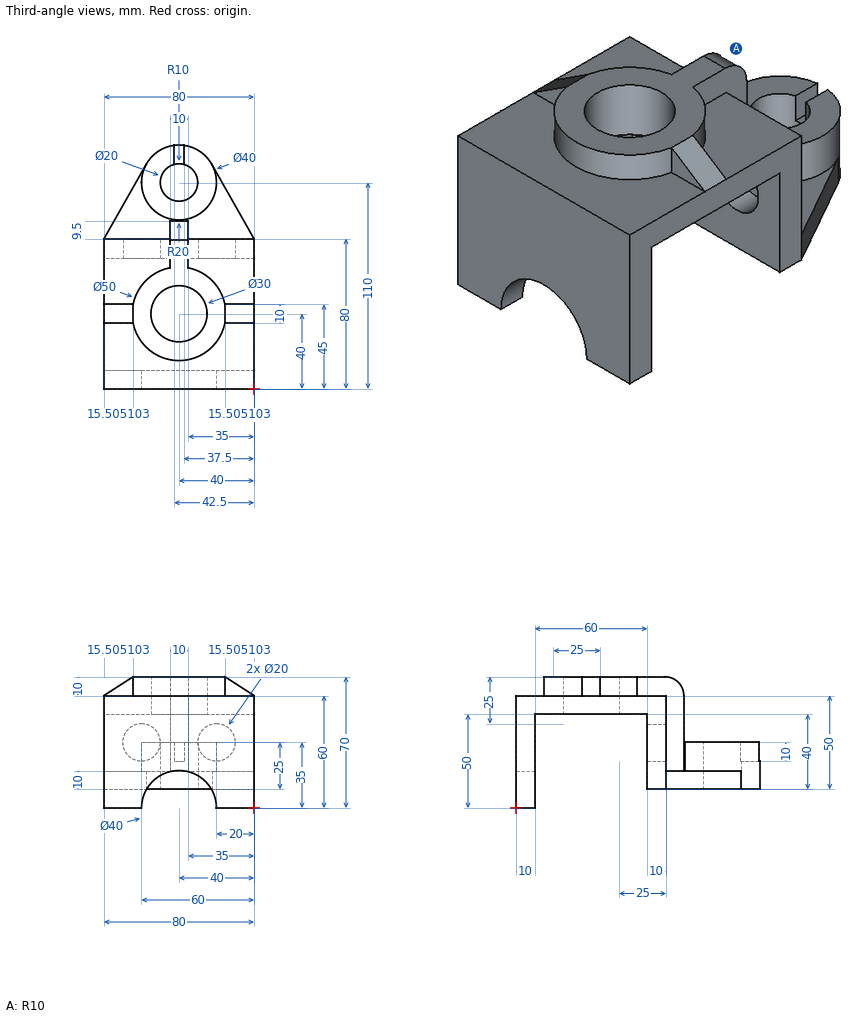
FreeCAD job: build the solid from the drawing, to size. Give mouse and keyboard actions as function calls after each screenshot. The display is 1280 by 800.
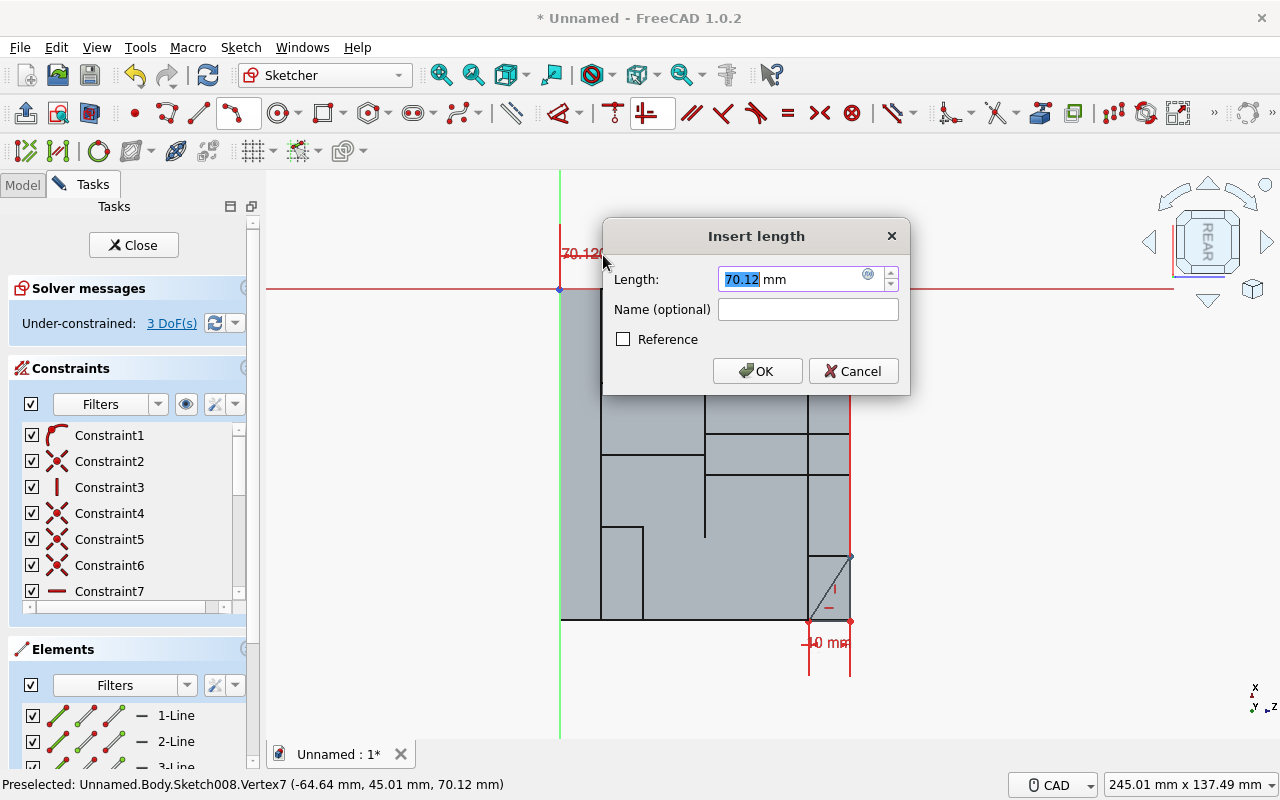
text(70)
key(Return)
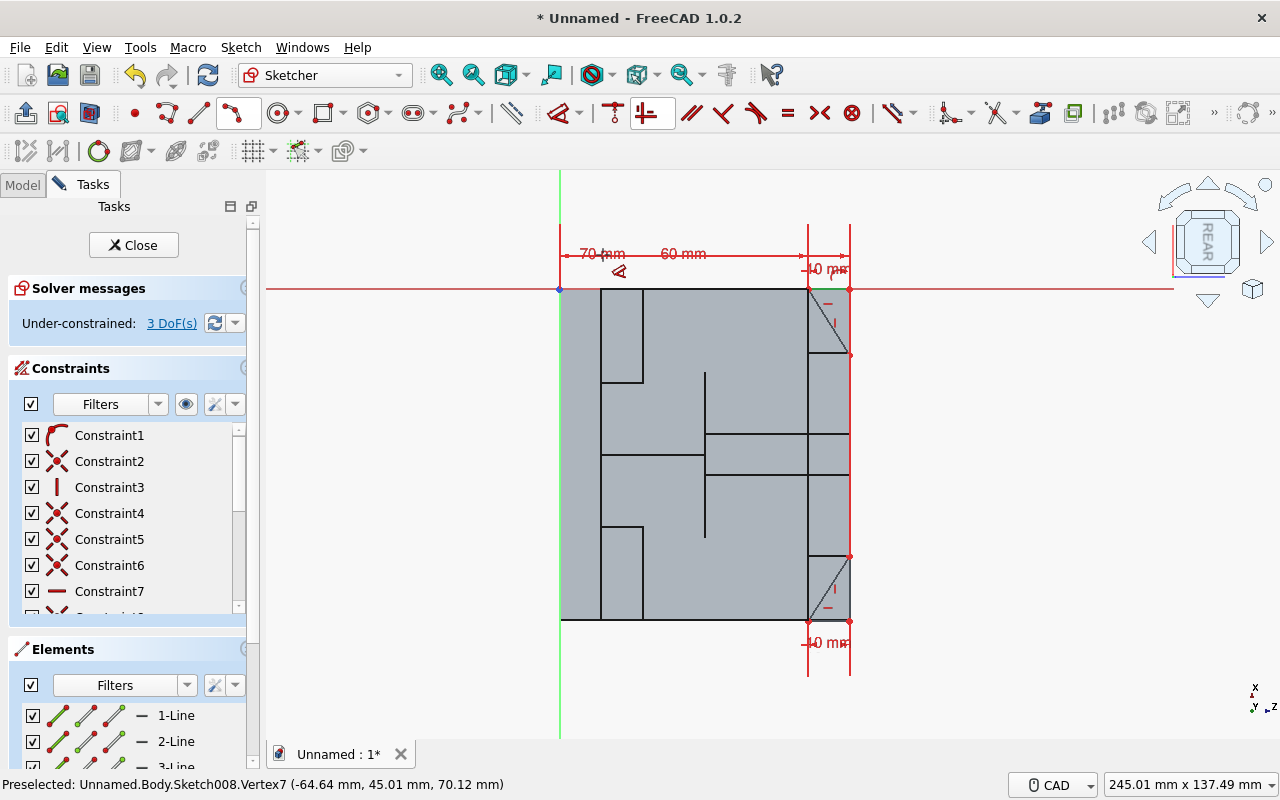
click(808, 621)
click(526, 455)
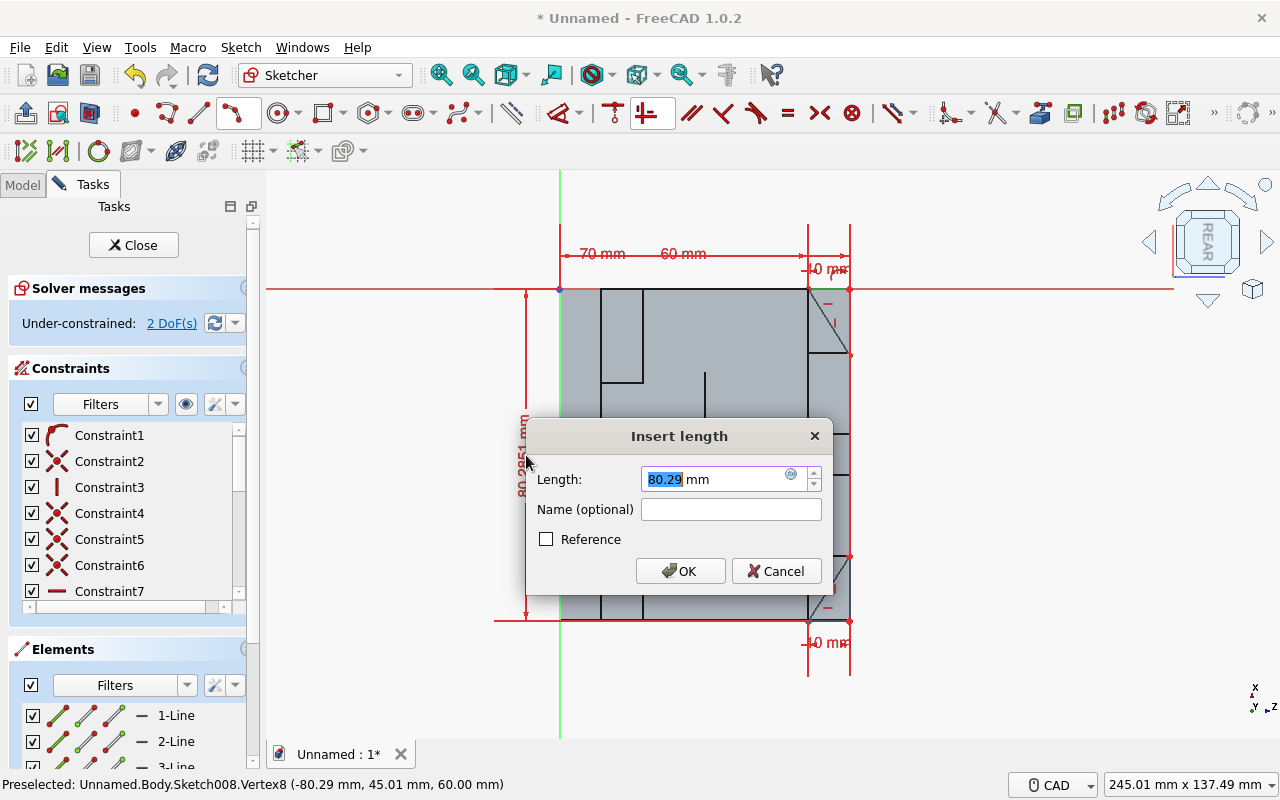
text(80)
key(Return)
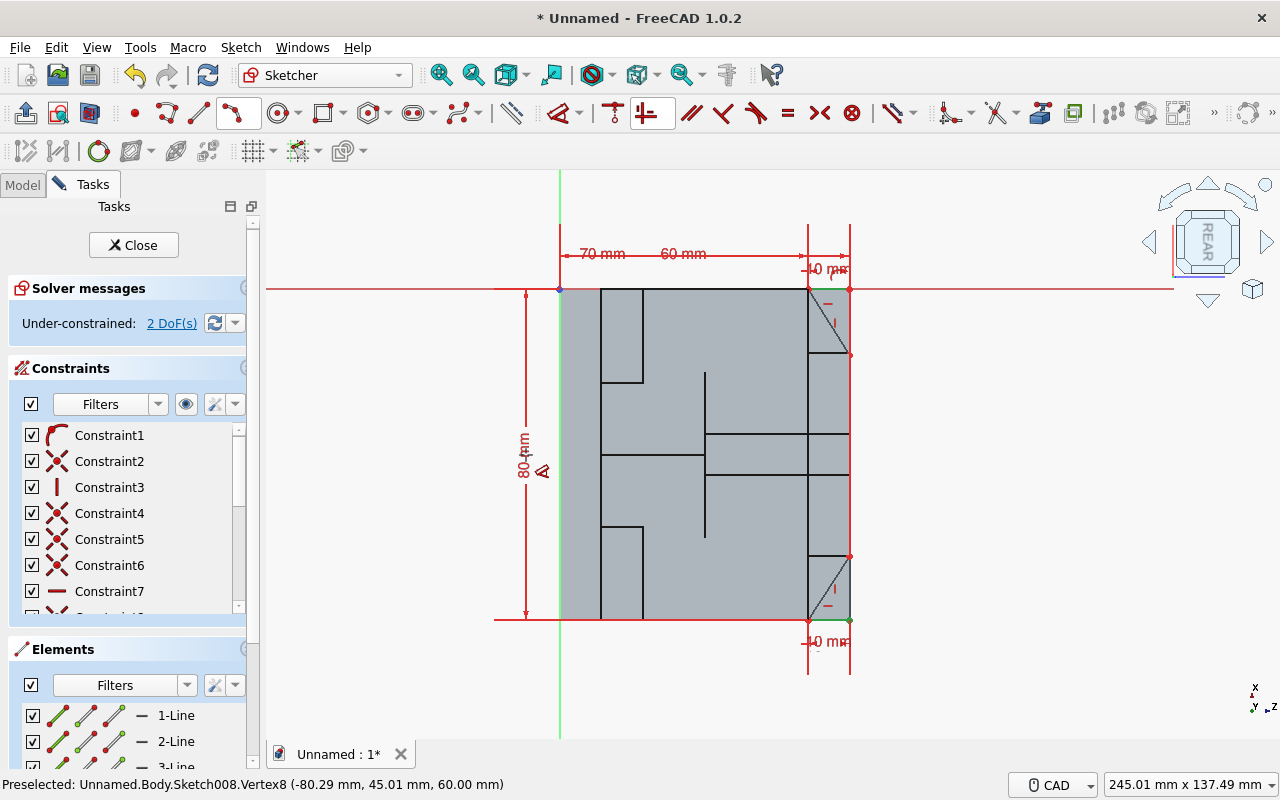
scroll(850, 335, up, 2)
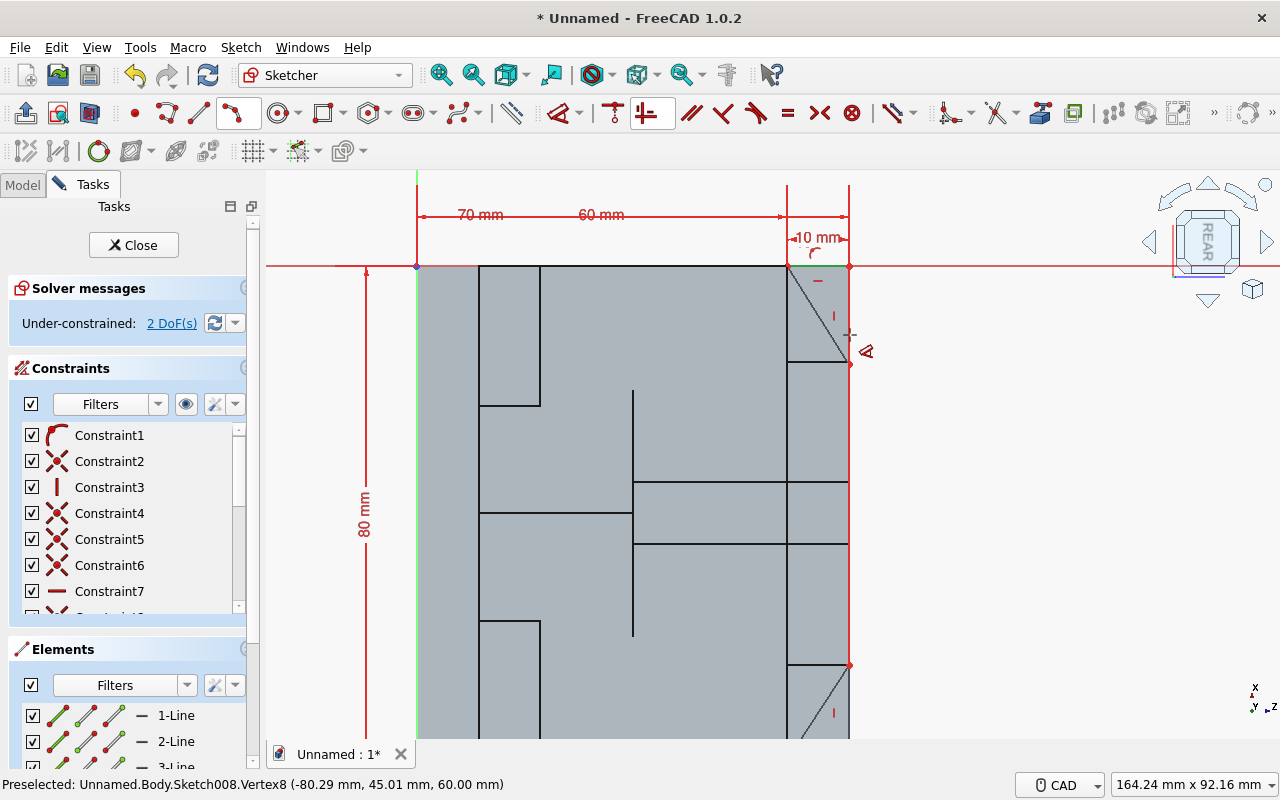
click(849, 335)
click(883, 316)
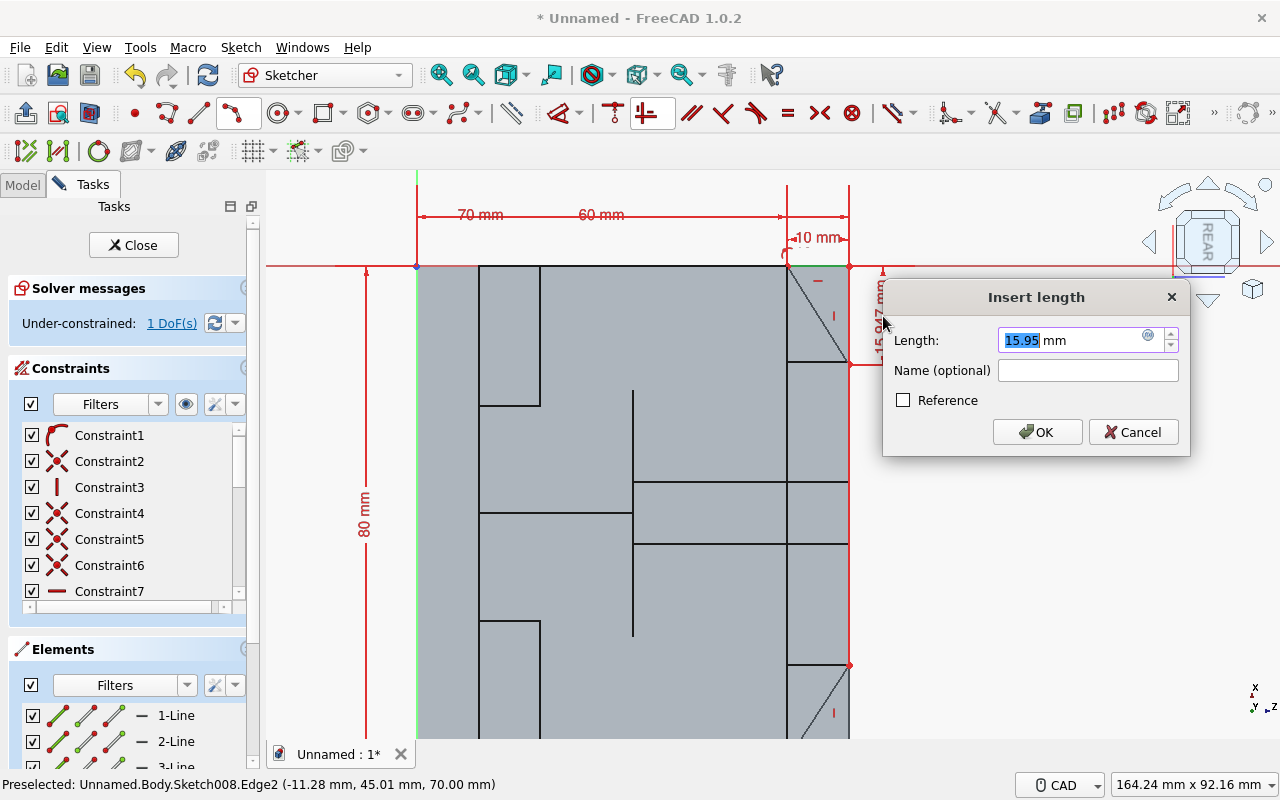
text(15.505103)
key(Return)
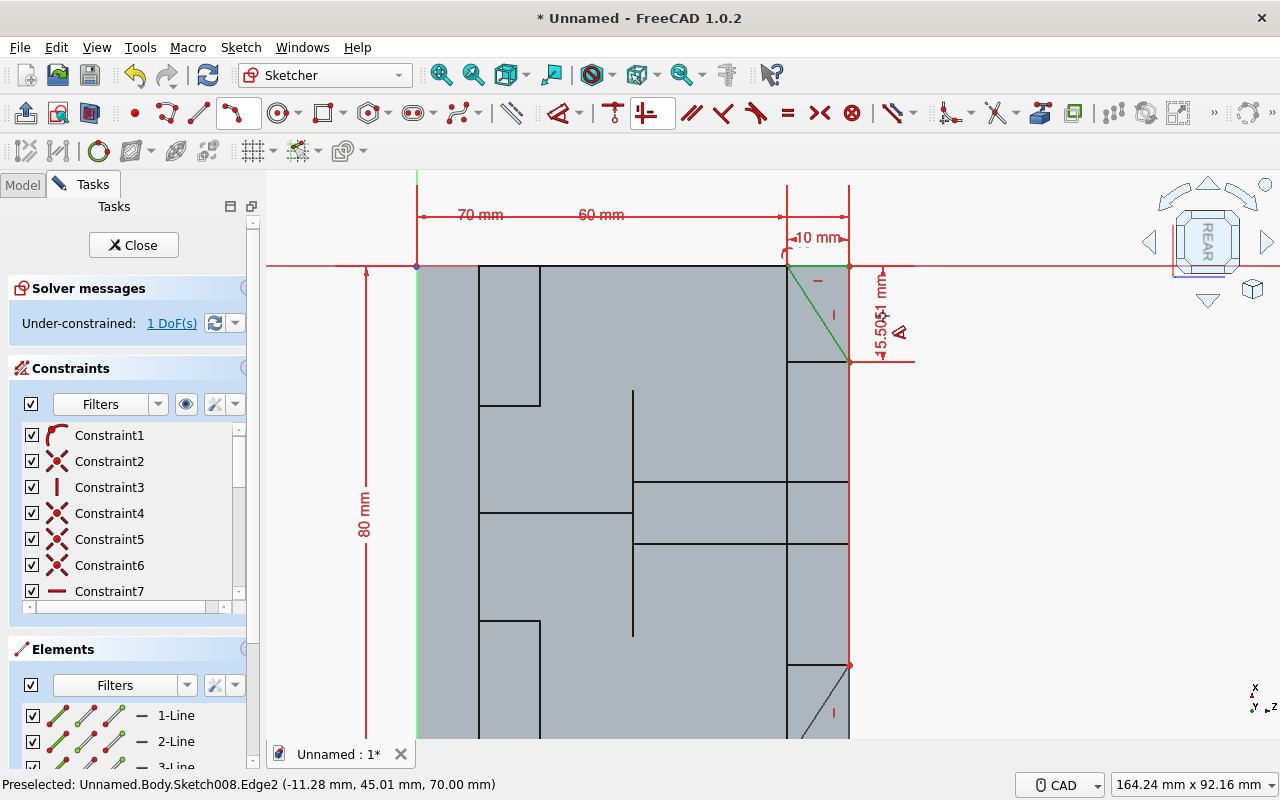
click(849, 694)
click(883, 688)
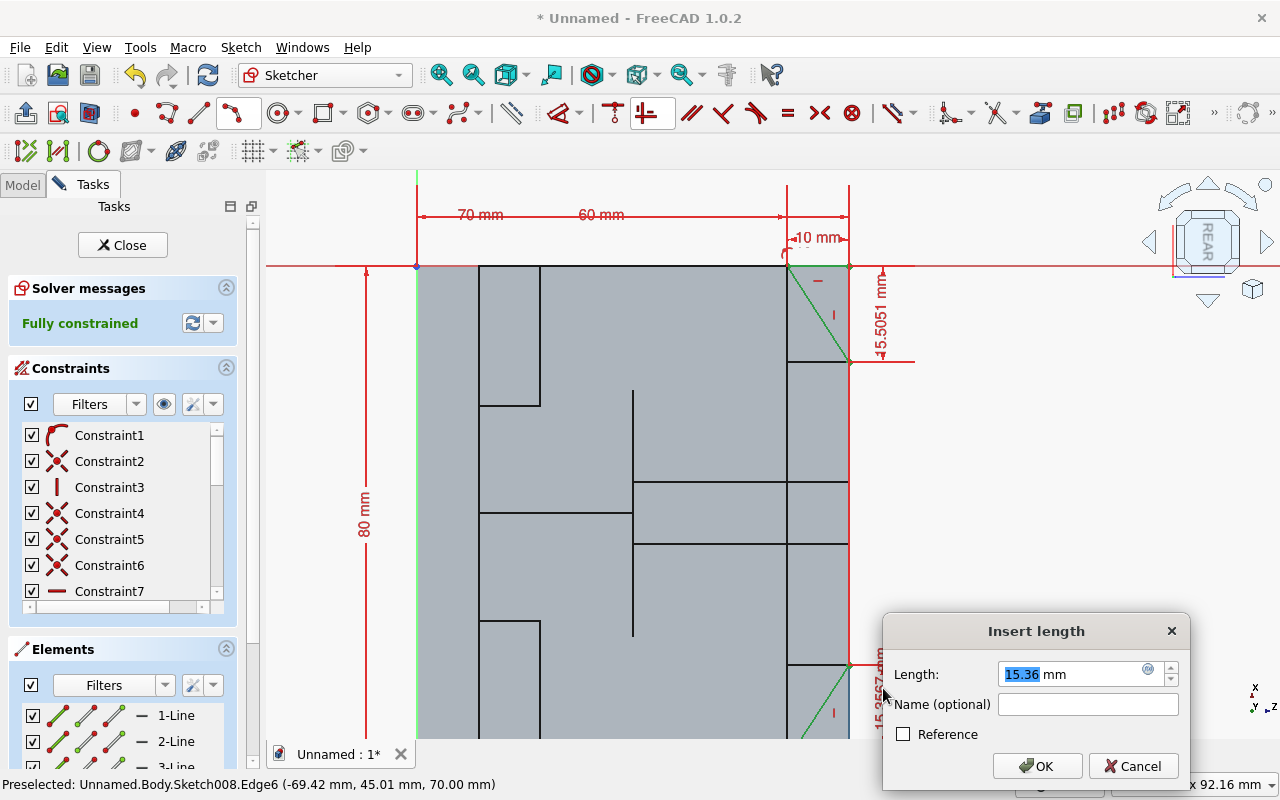
text(15.505103)
key(Return)
key(Escape)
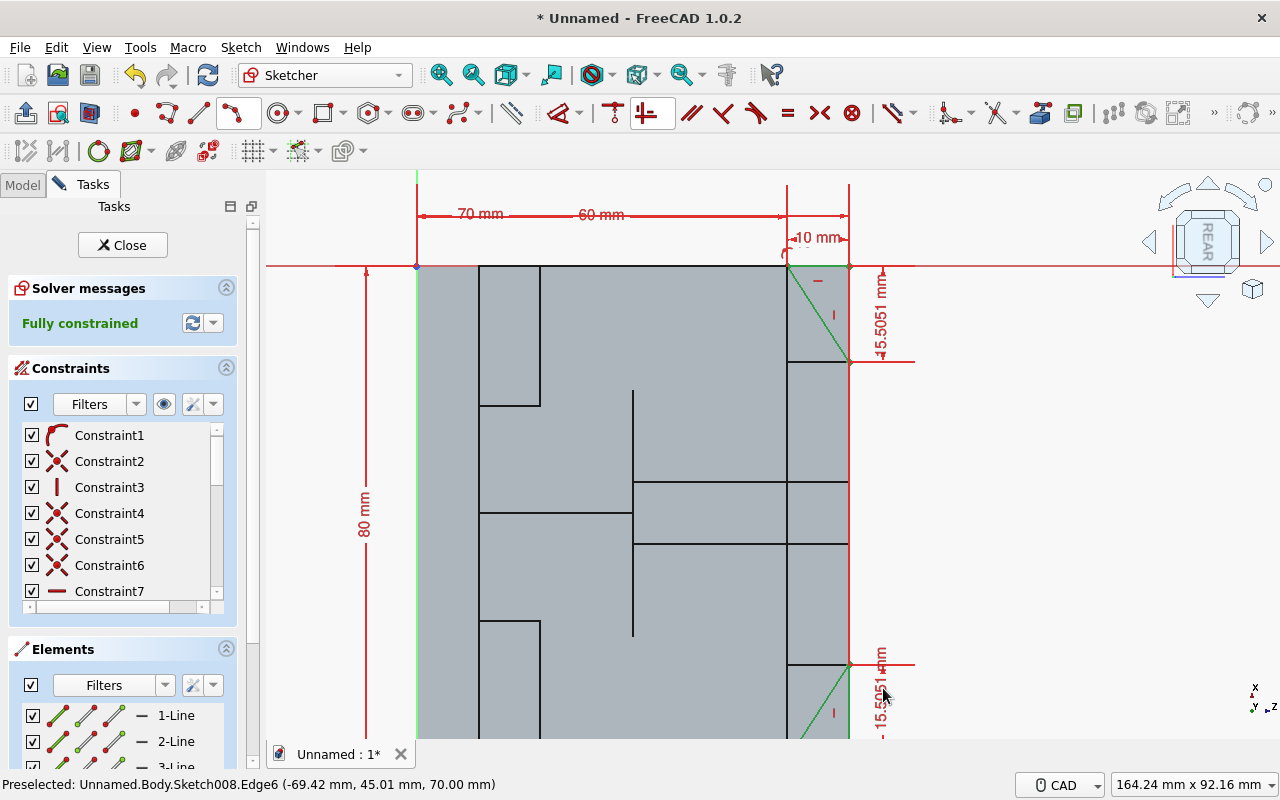
click(123, 245)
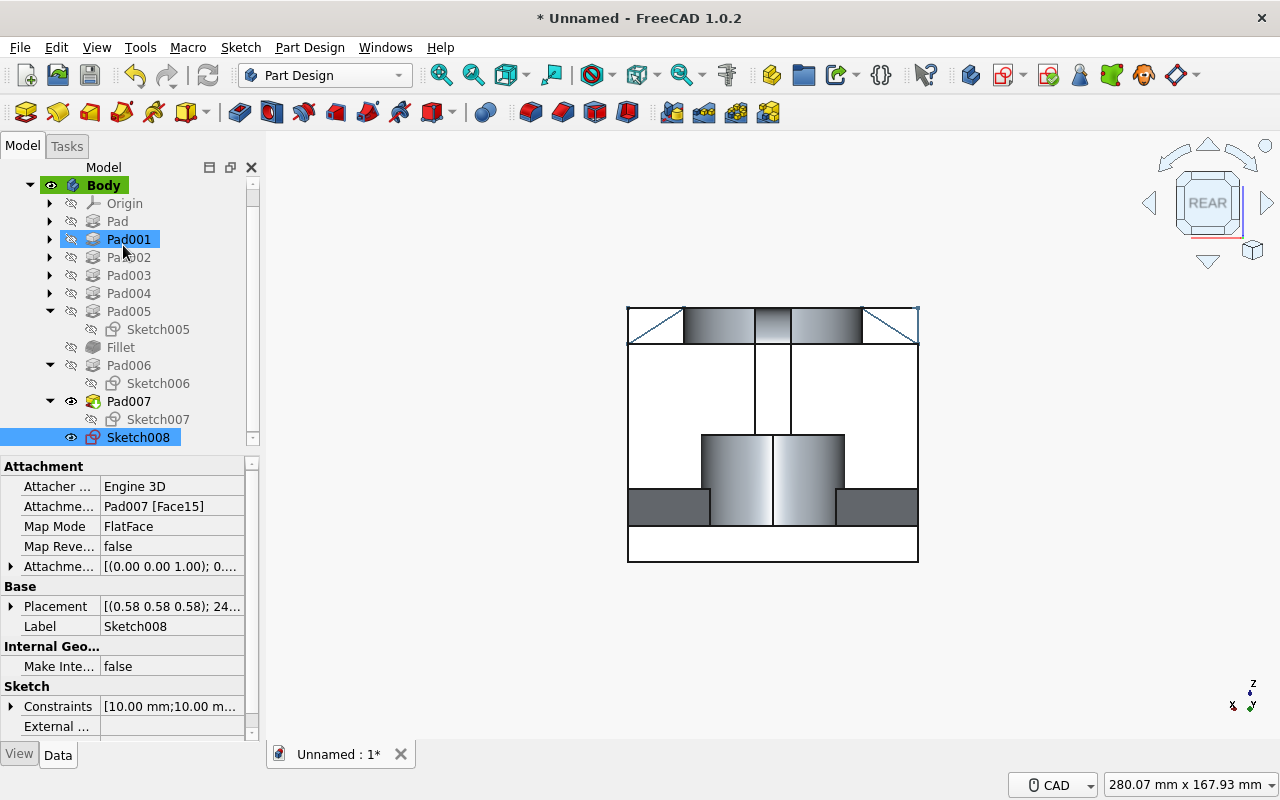
click(240, 112)